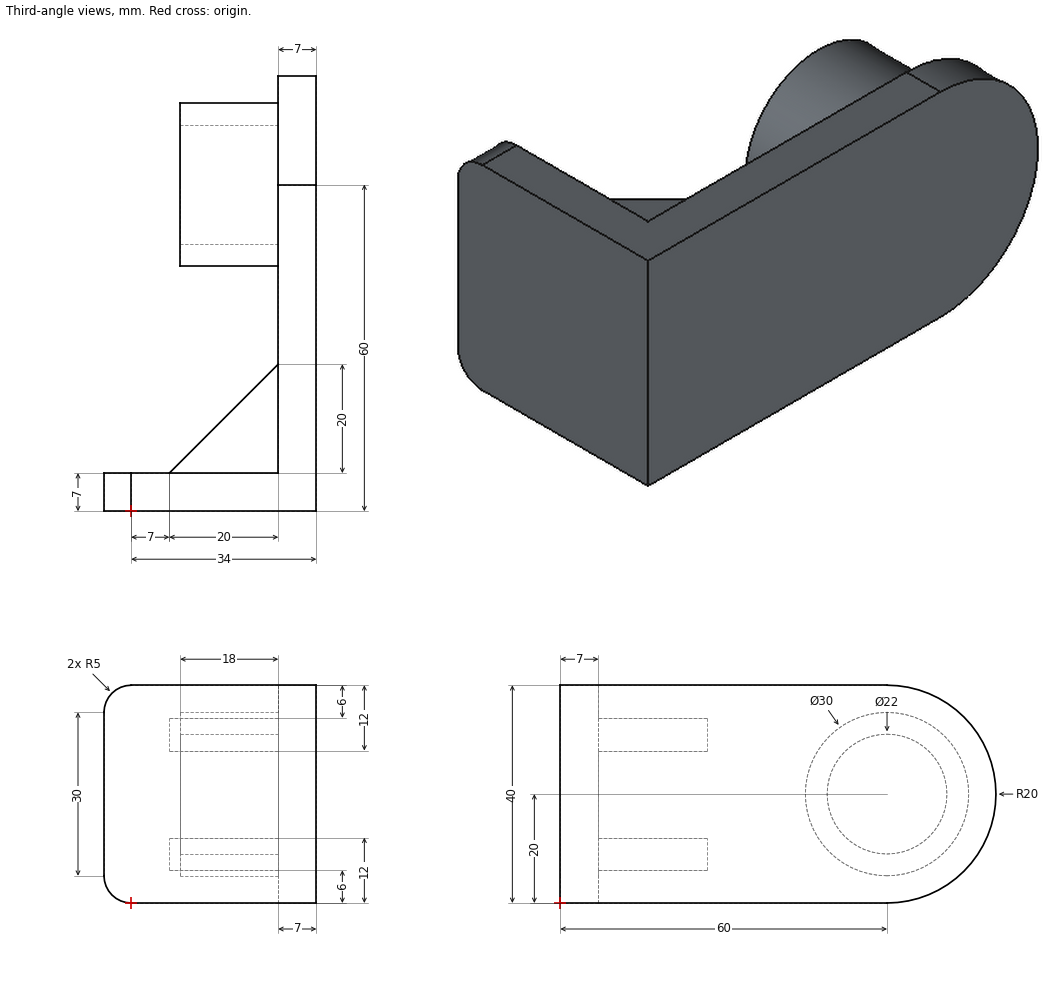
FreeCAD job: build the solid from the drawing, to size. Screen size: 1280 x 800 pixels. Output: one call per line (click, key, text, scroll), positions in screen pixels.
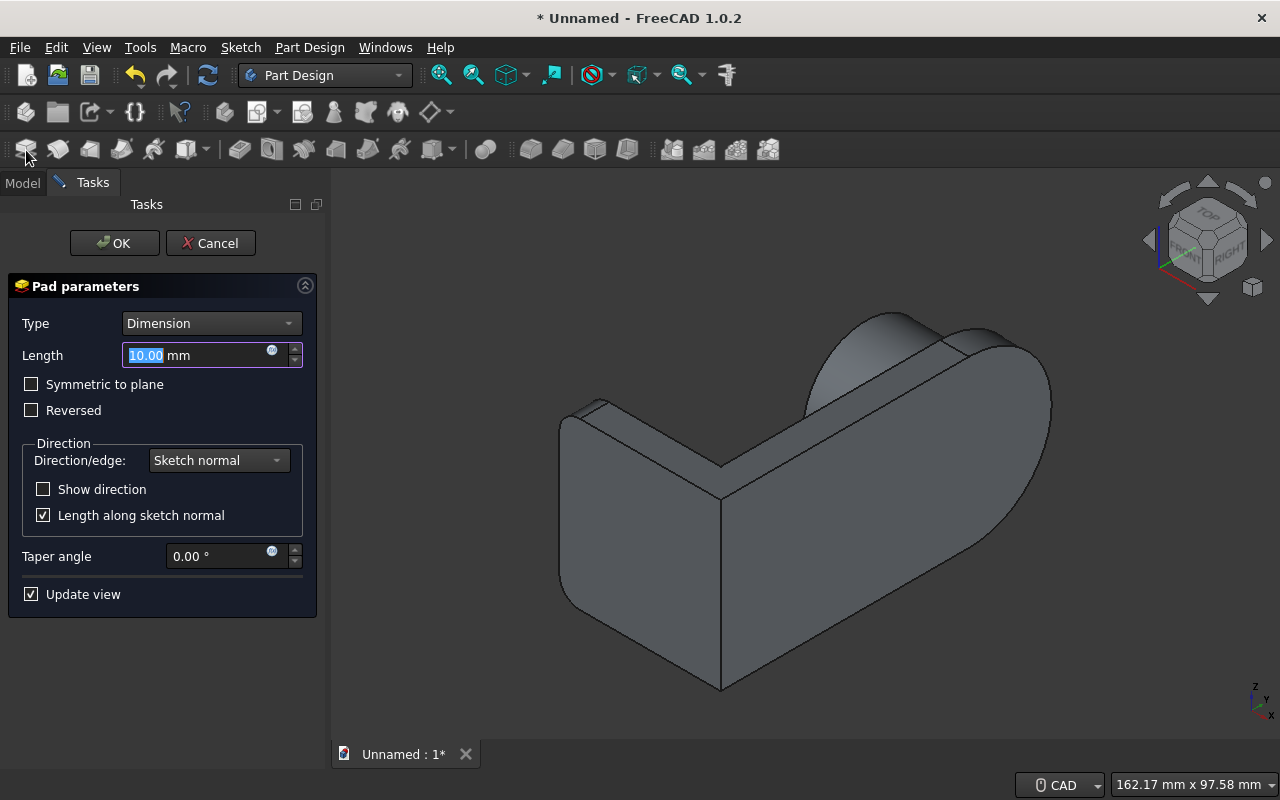
text(12)
key(Tab)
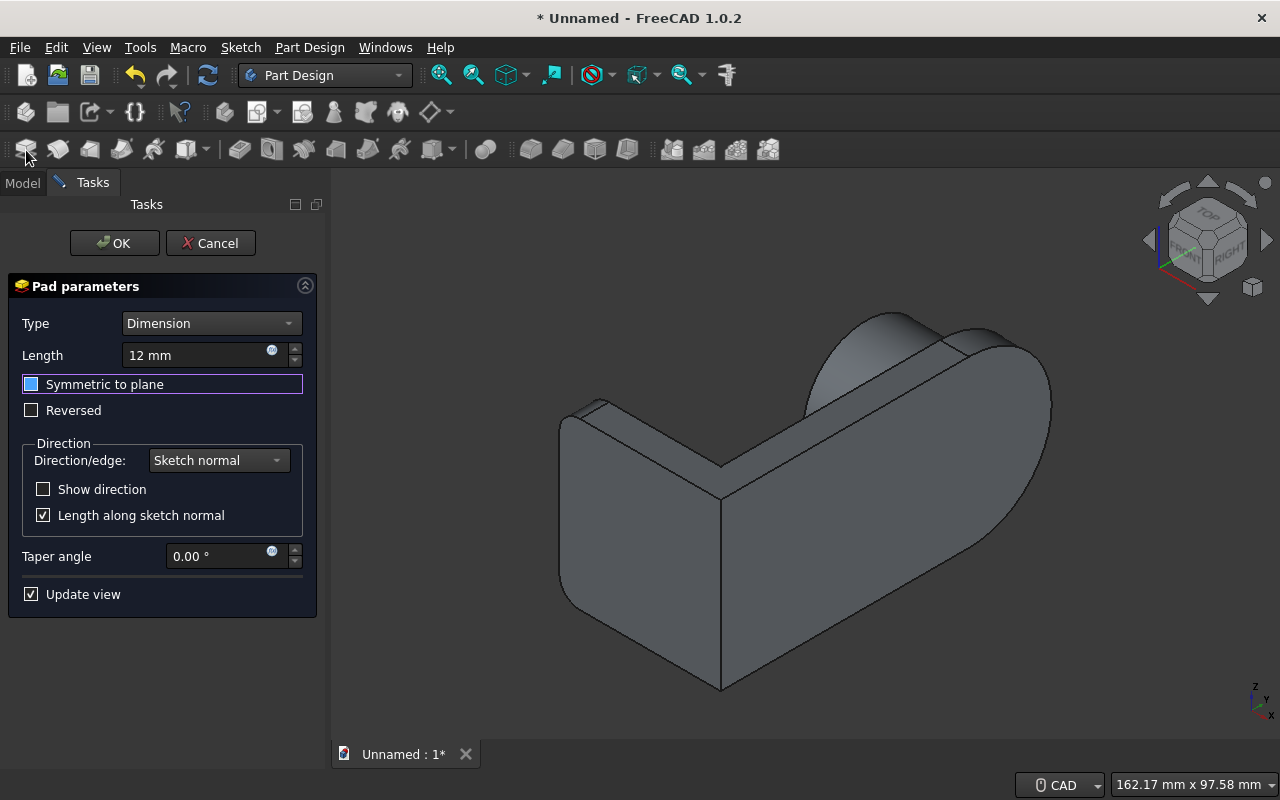
click(30, 410)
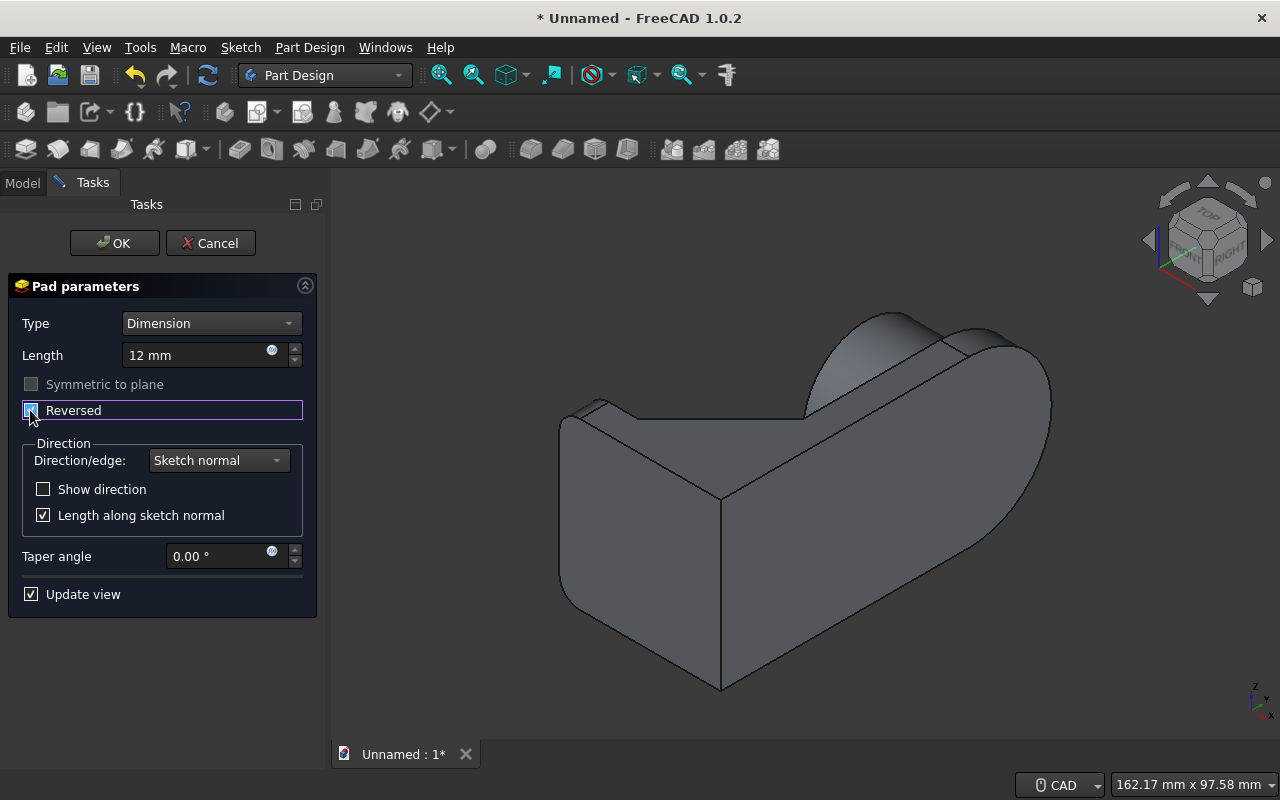
click(115, 243)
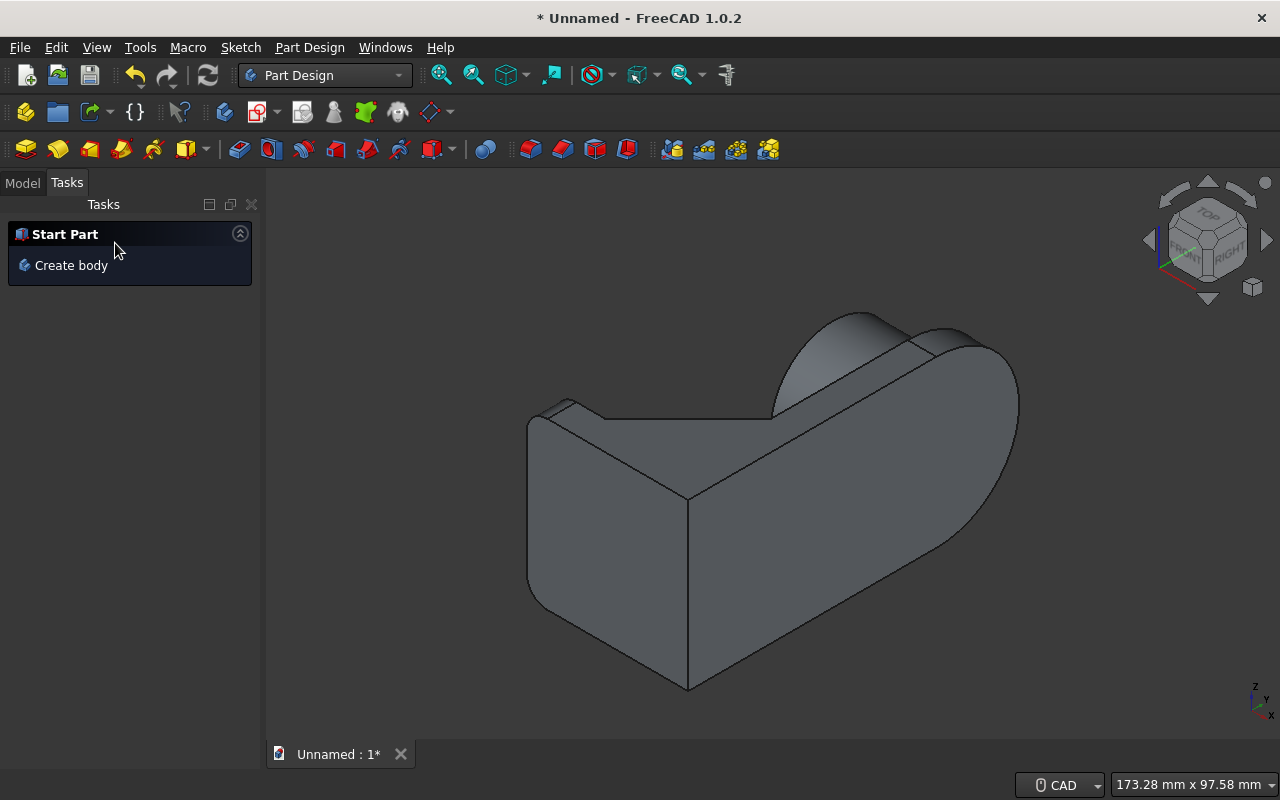
click(258, 112)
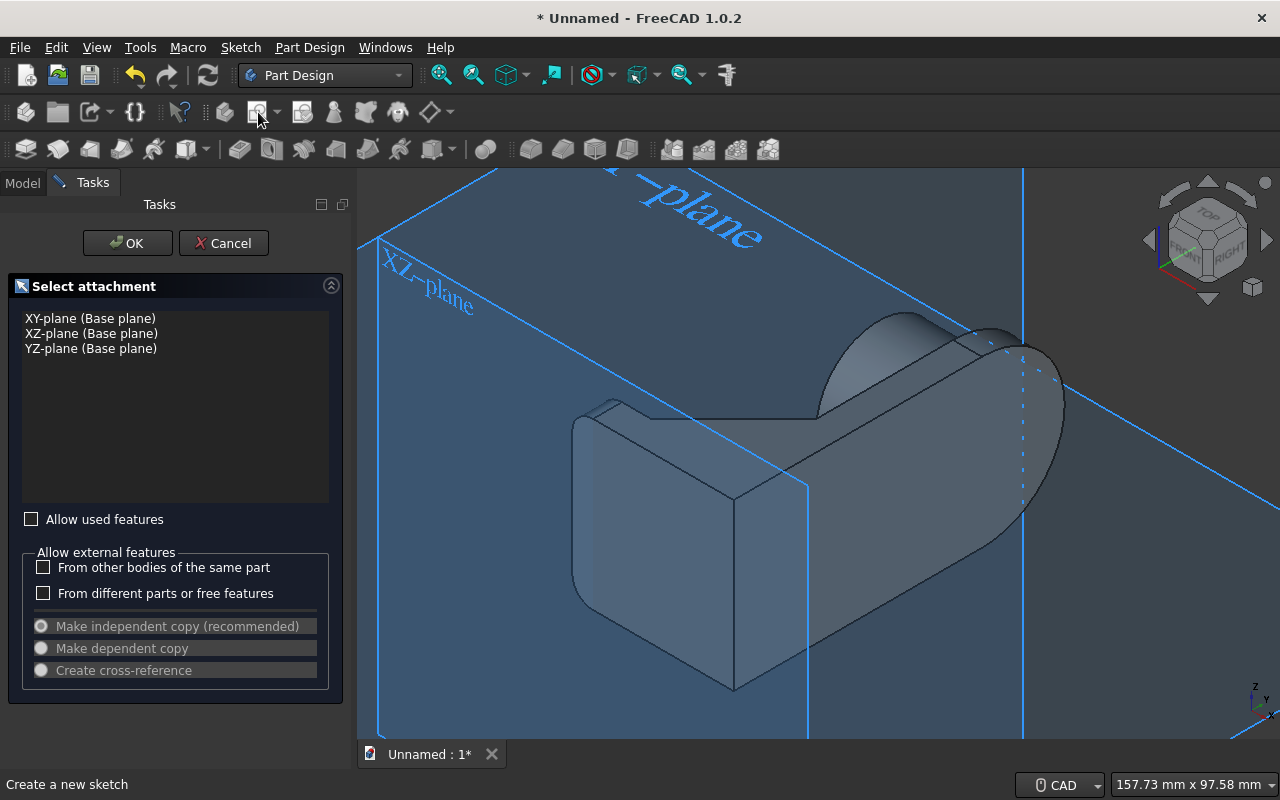
click(82, 318)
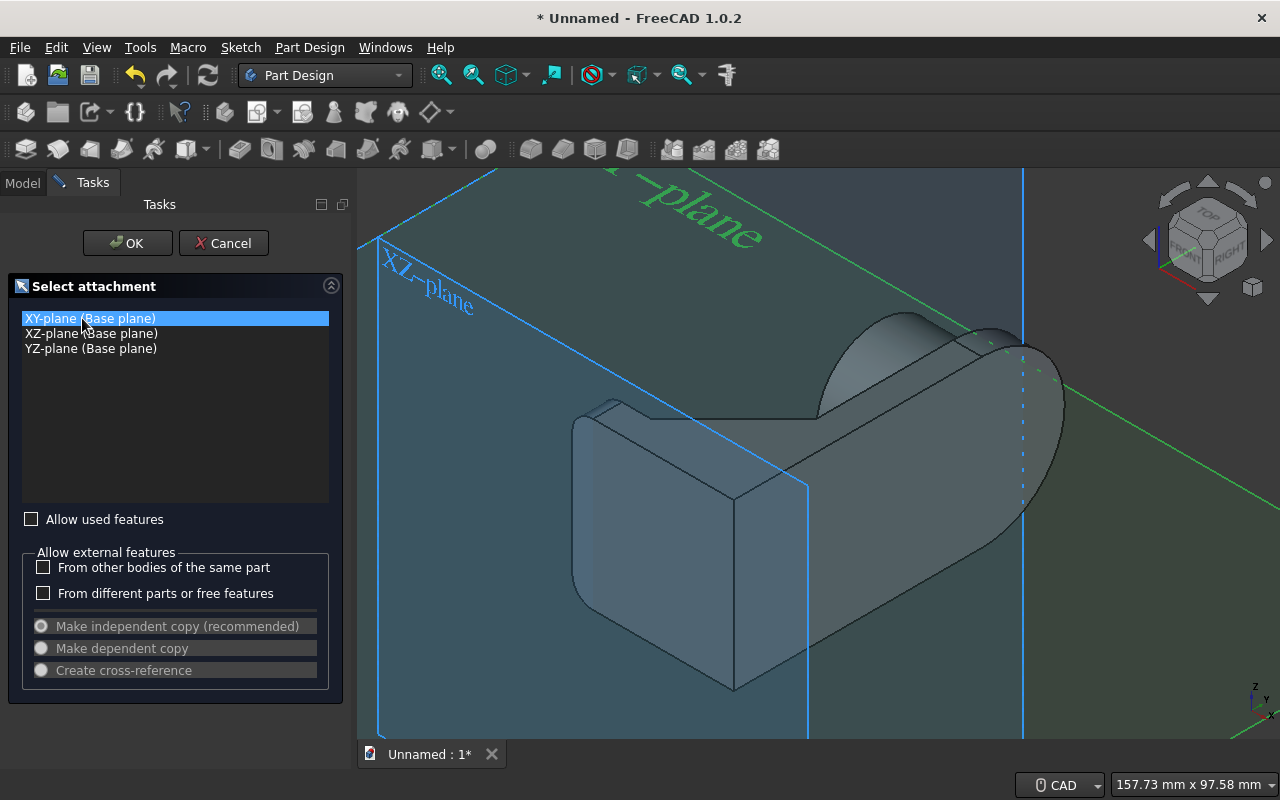
click(128, 243)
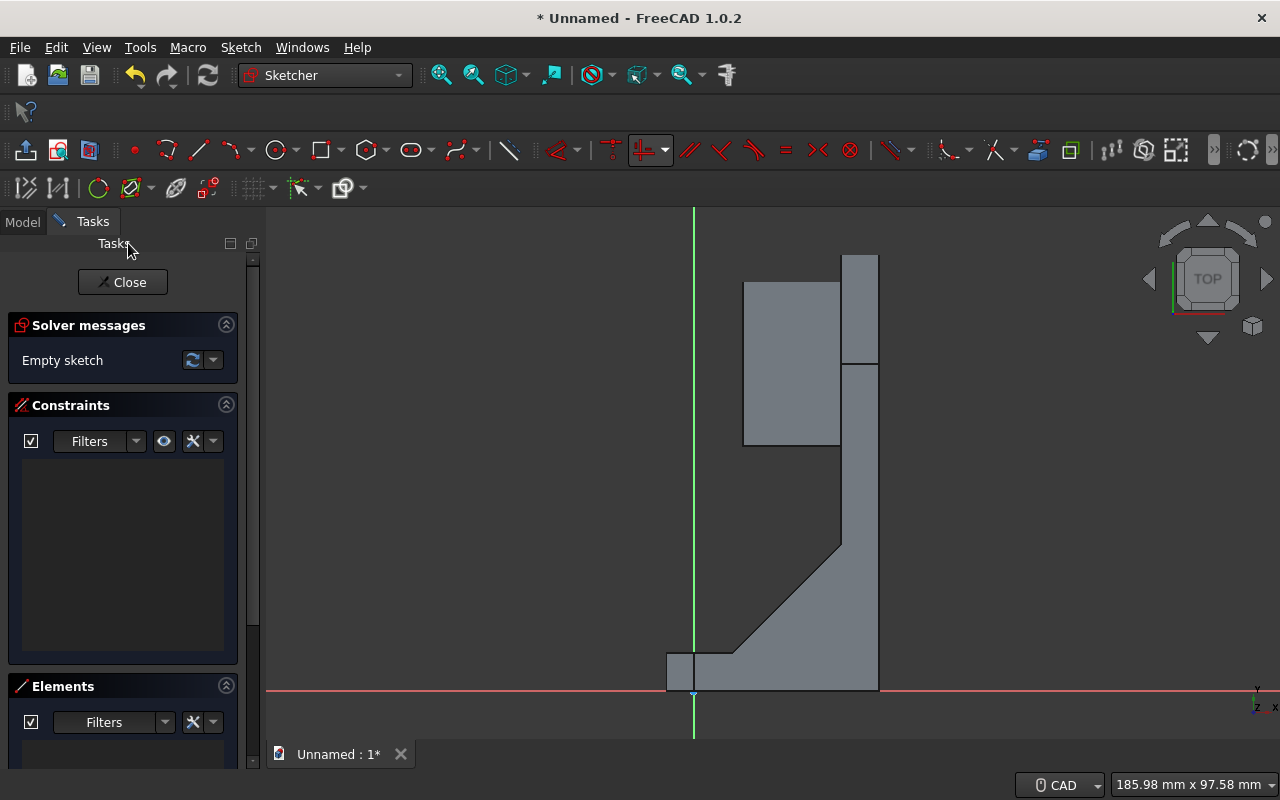
click(90, 150)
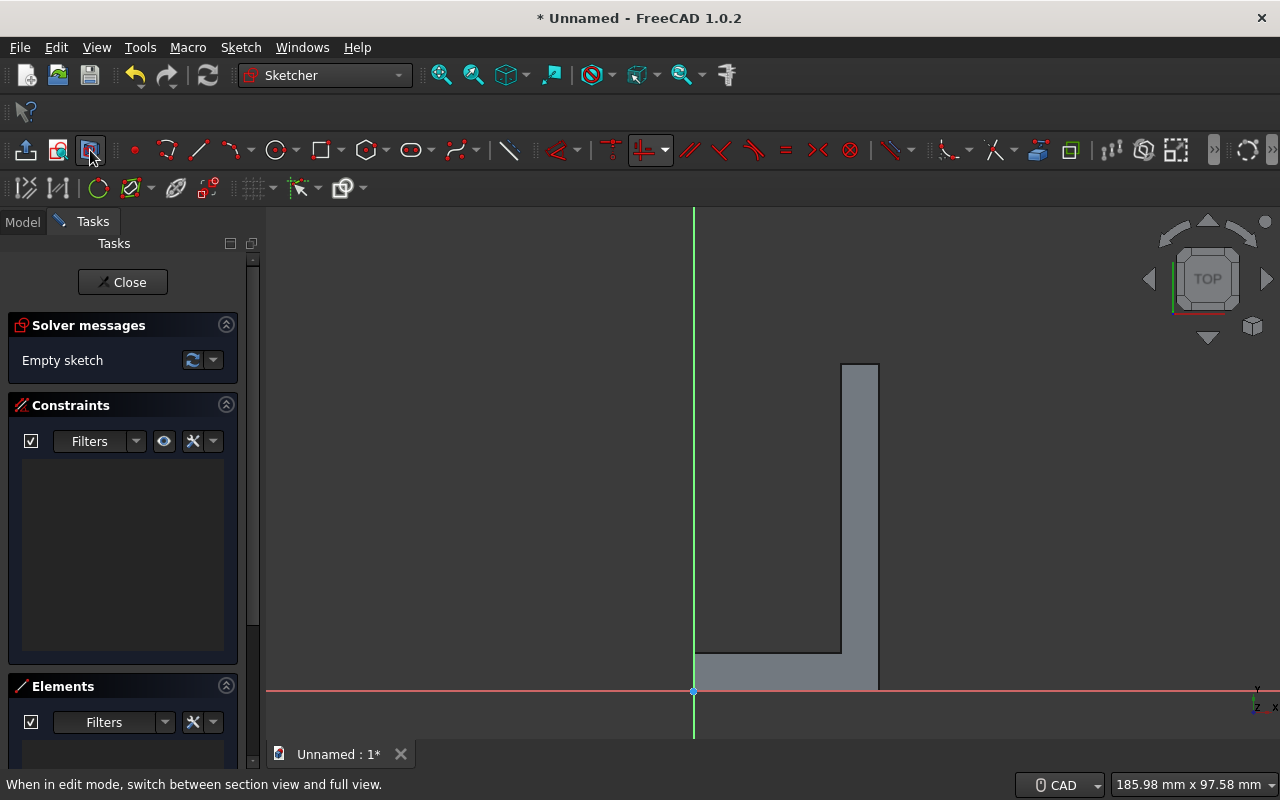
scroll(819, 711, up, 4)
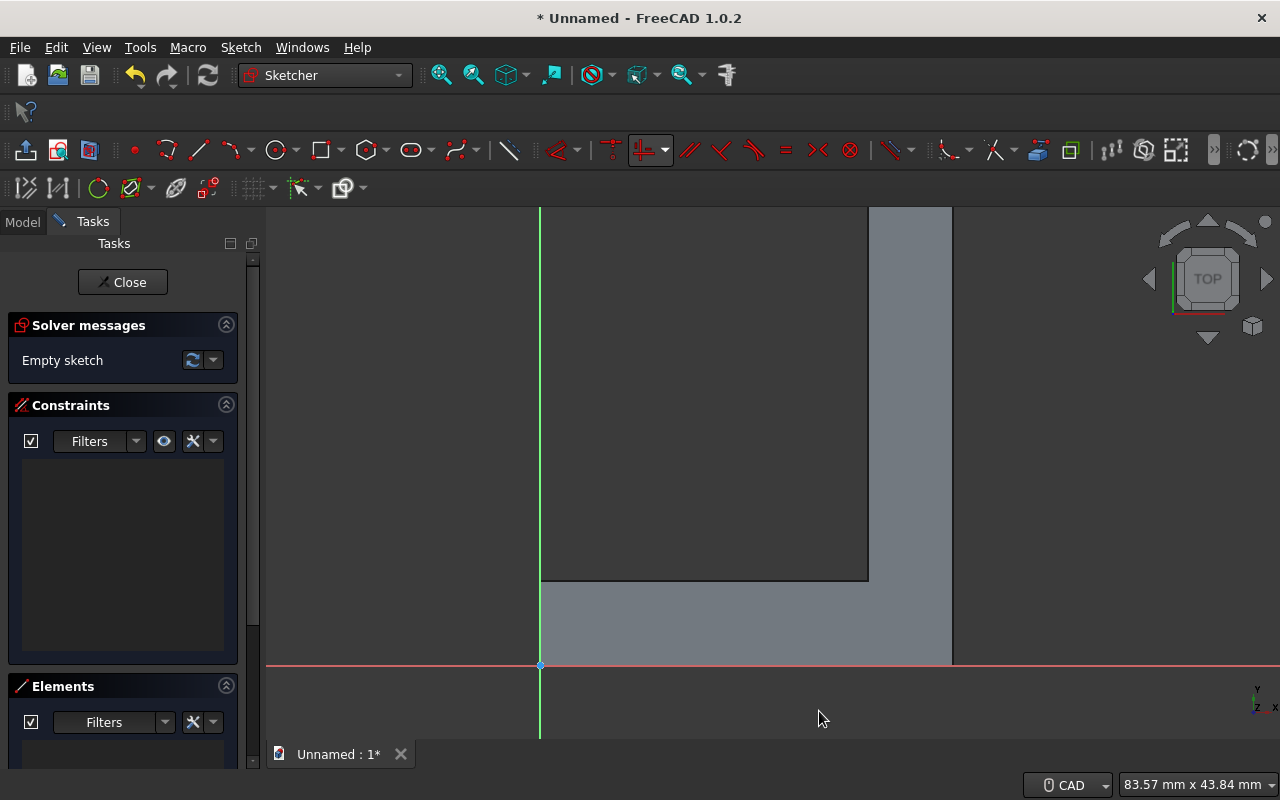
click(168, 150)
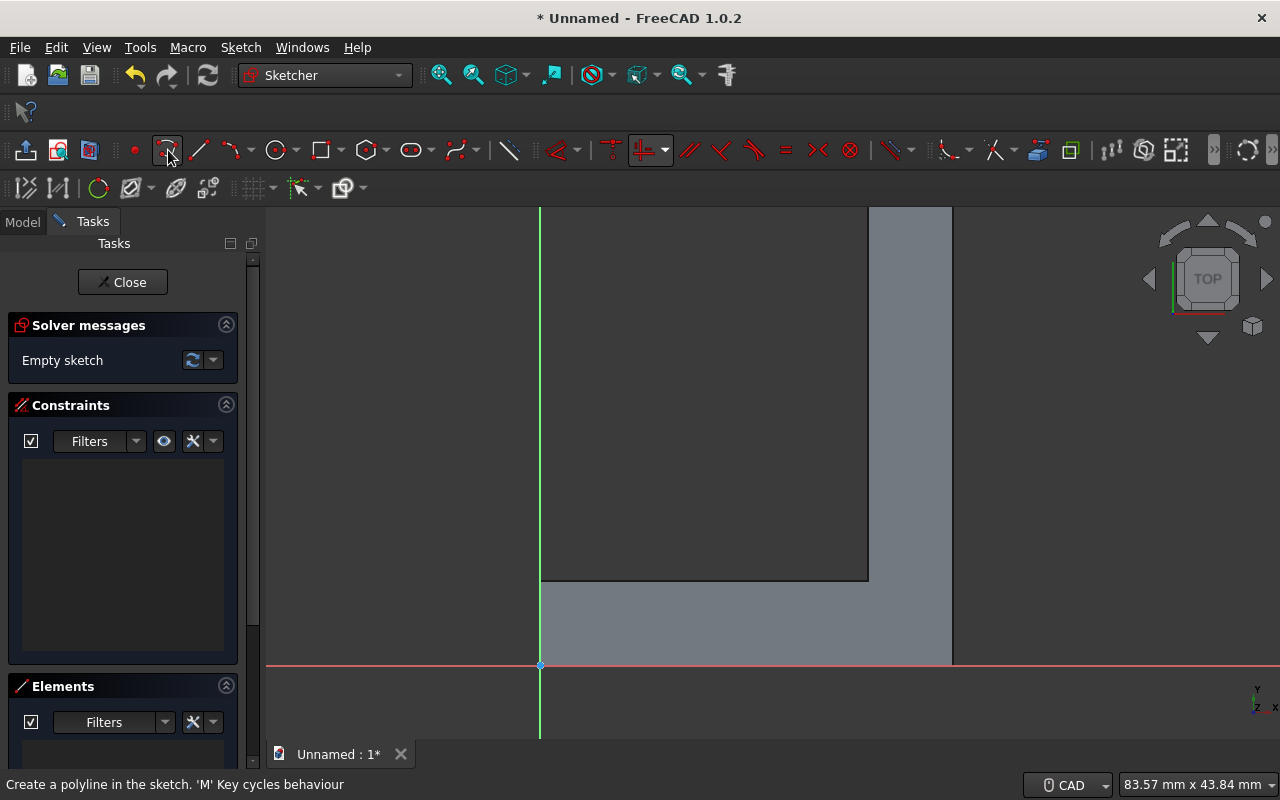
click(625, 581)
click(868, 338)
click(868, 581)
click(625, 582)
key(Escape)
key(Escape)